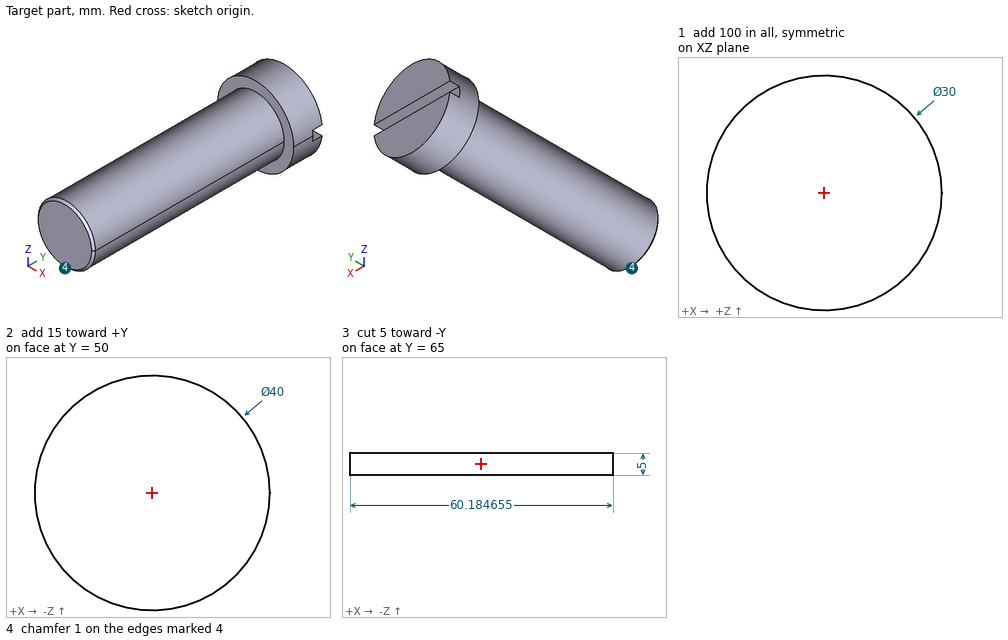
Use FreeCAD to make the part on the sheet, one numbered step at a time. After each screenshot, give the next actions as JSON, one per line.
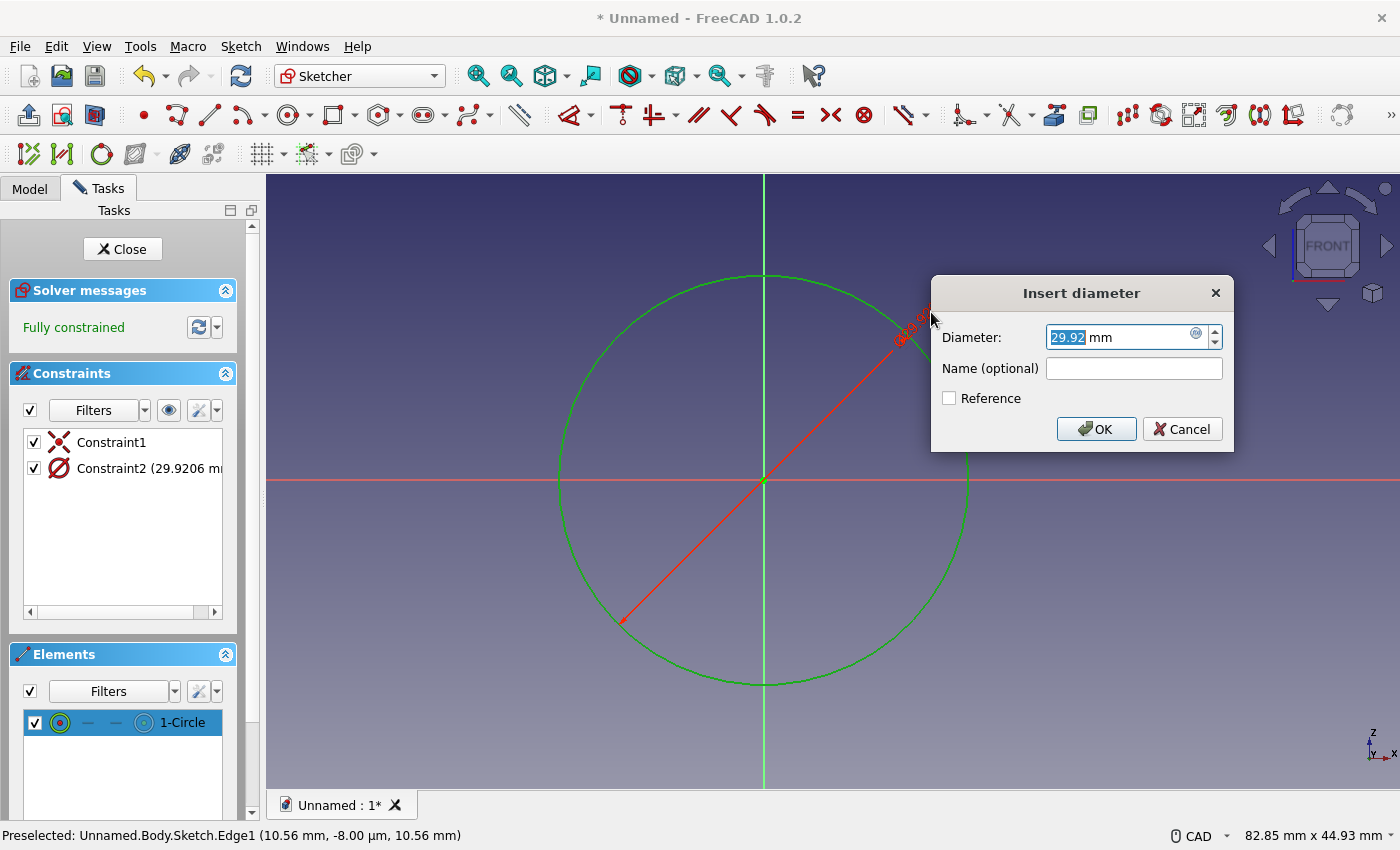
{"action": "type", "text": "30"}
{"action": "key", "text": "Return"}
{"action": "key", "text": "Escape"}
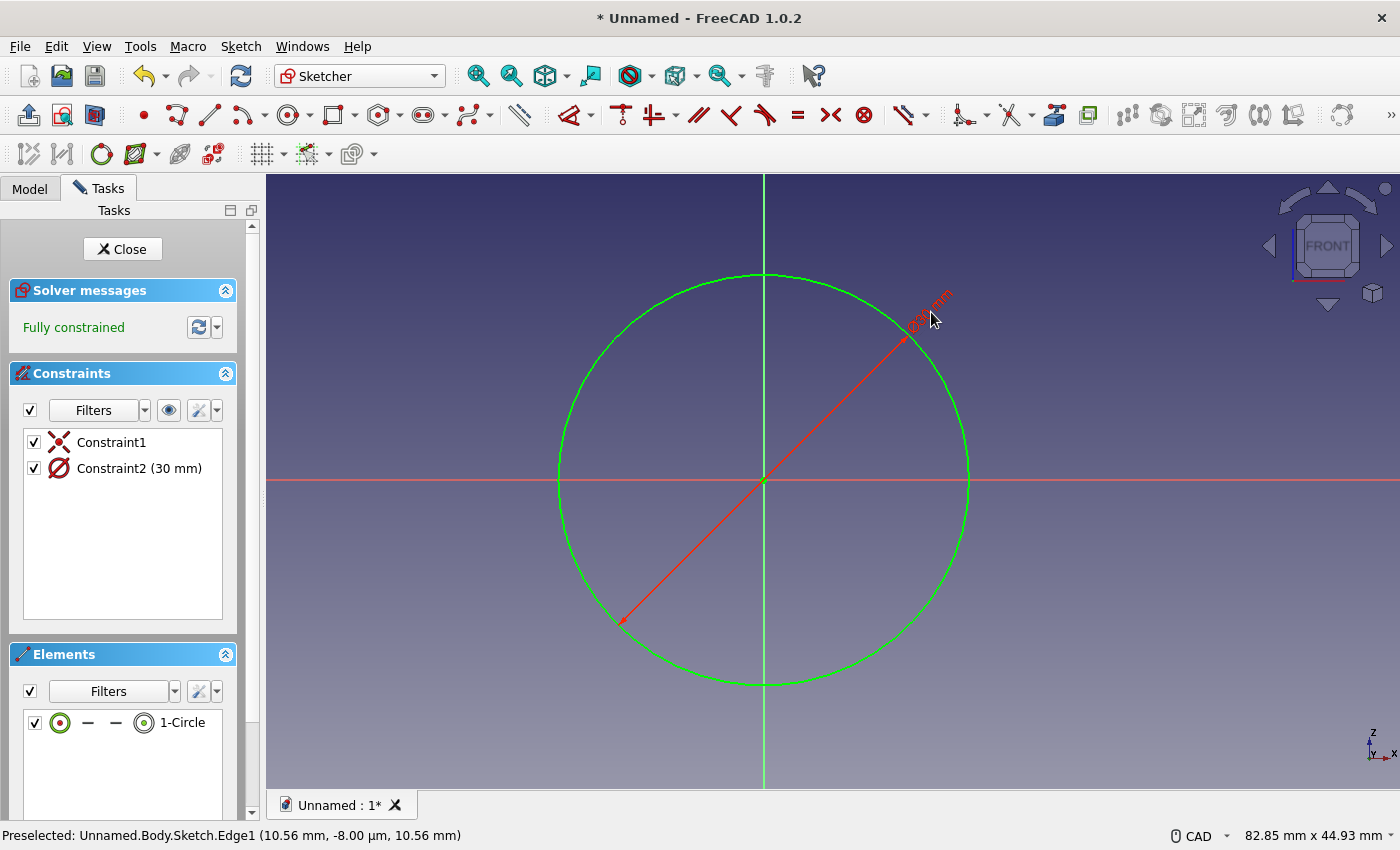
{"action": "left_click", "coordinate": [123, 249]}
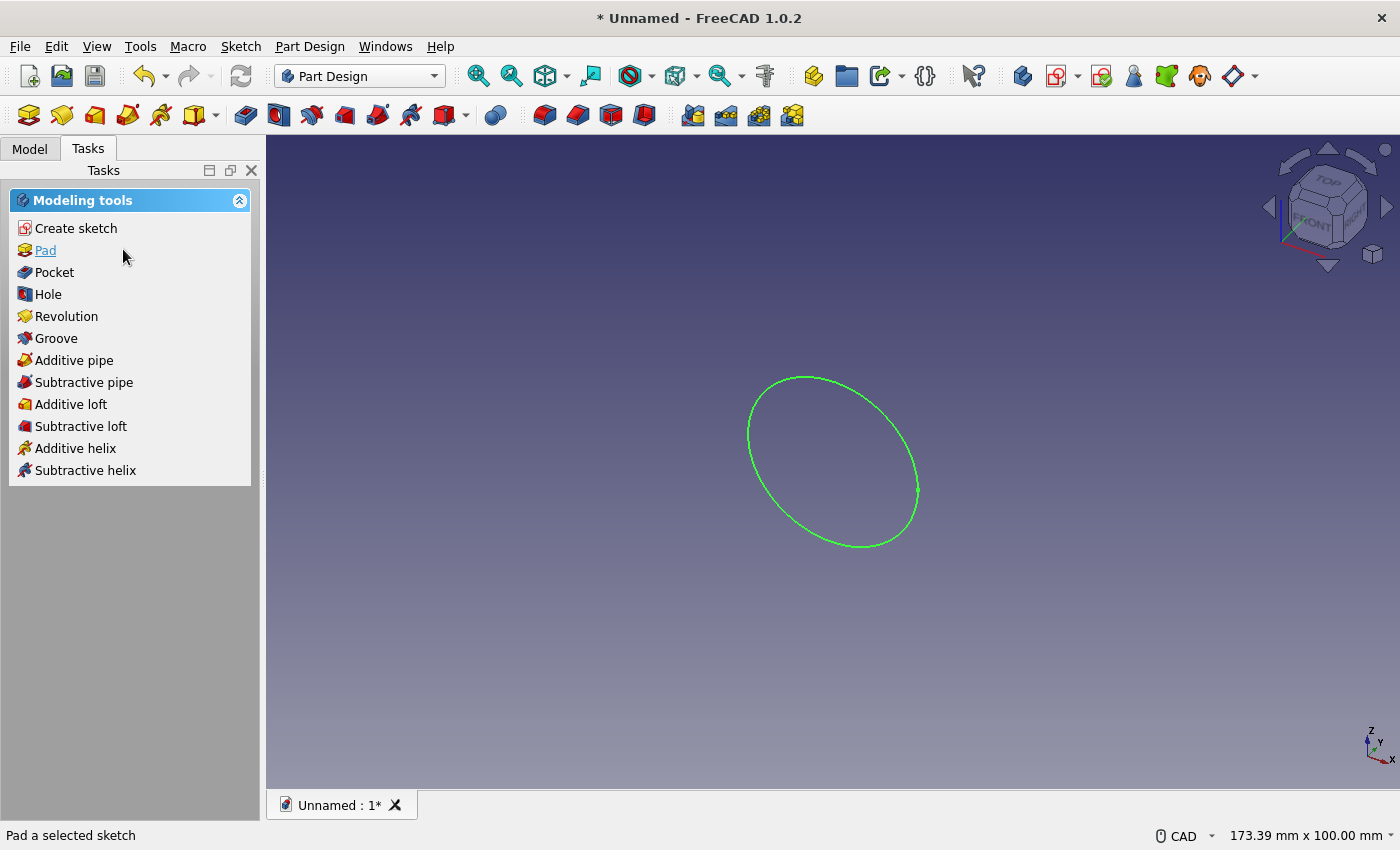
{"action": "left_click", "coordinate": [29, 116]}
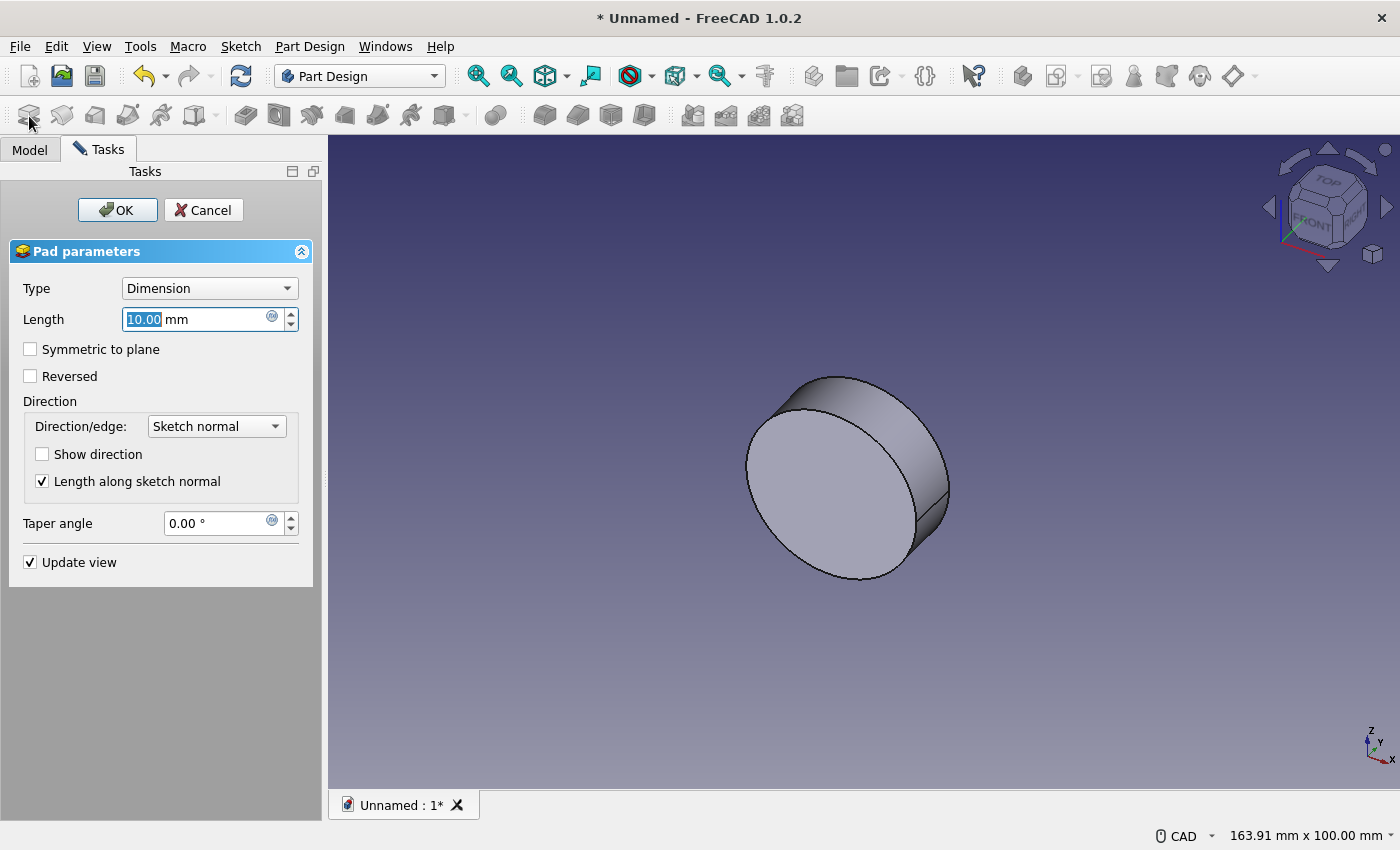
{"action": "type", "text": "100"}
{"action": "key", "text": "Tab"}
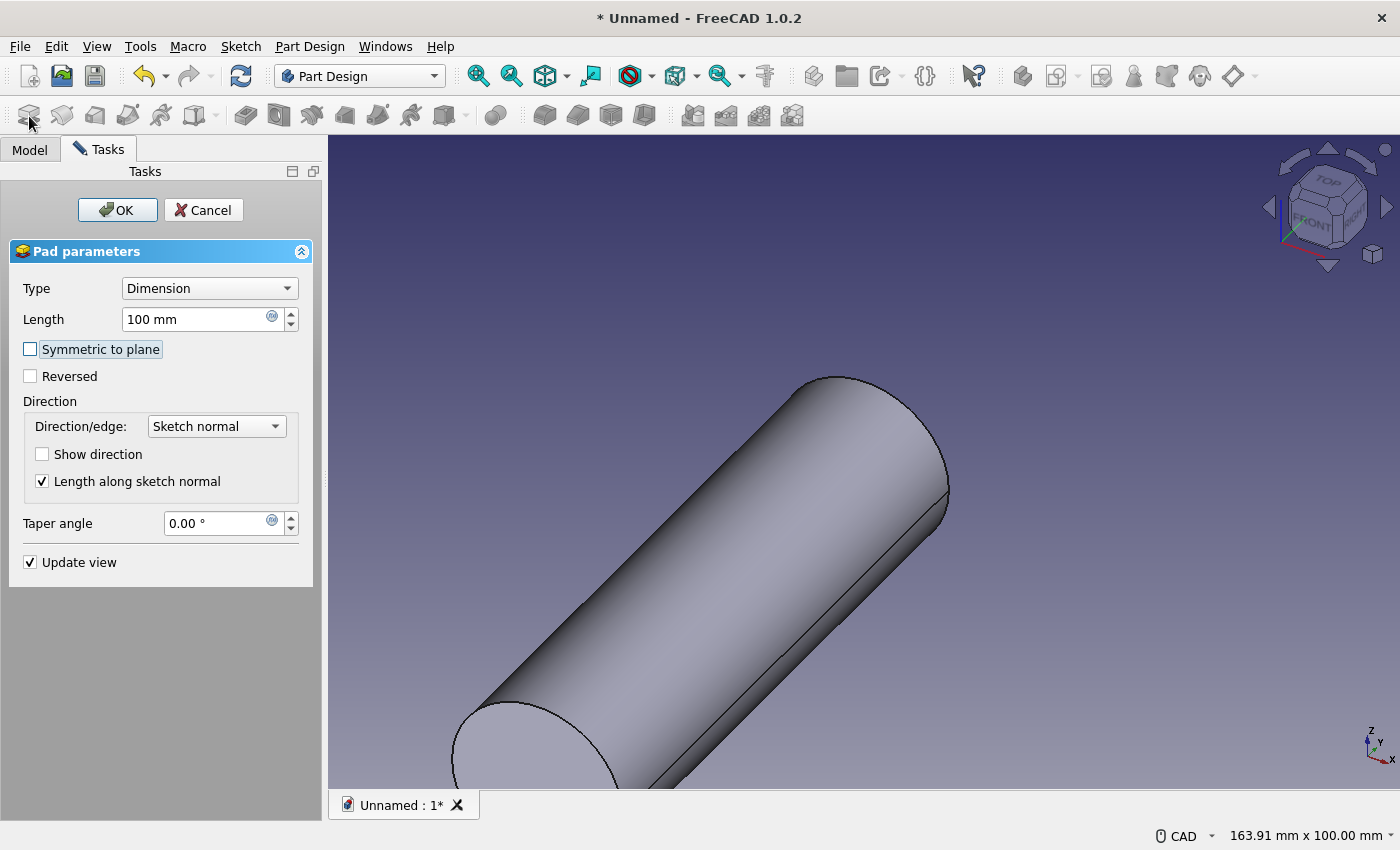
{"action": "left_click", "coordinate": [31, 349]}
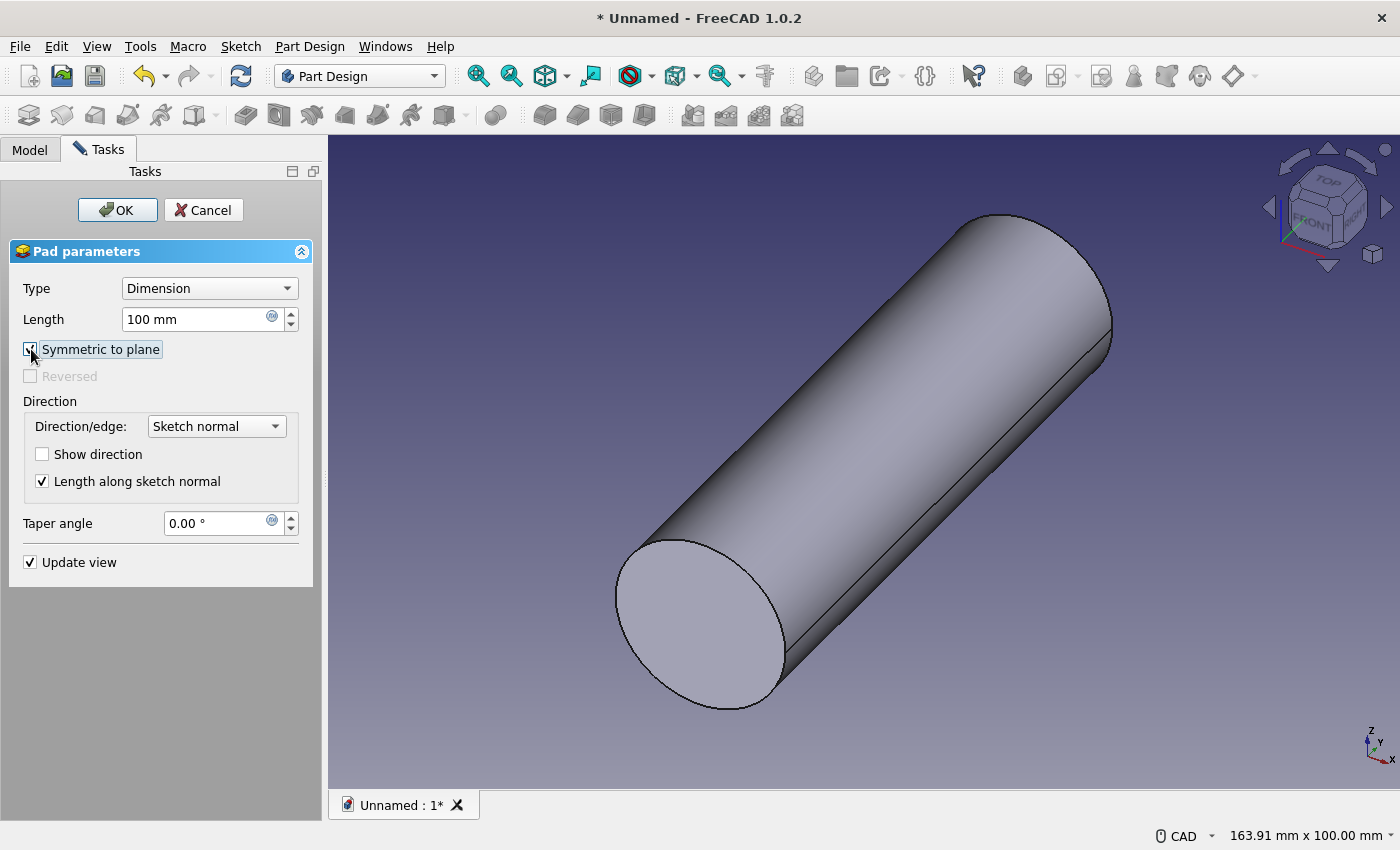
{"action": "left_click", "coordinate": [118, 210]}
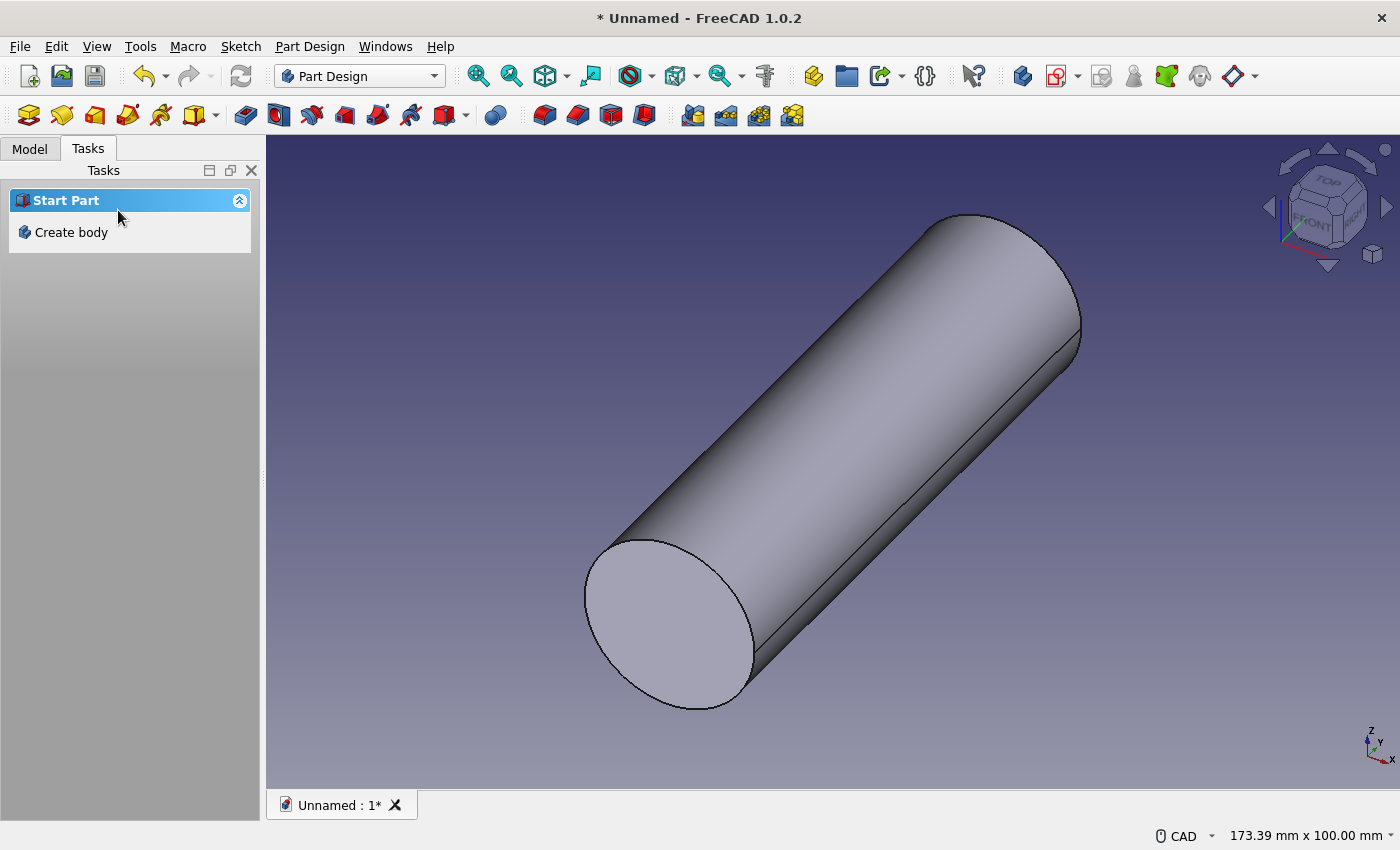
{"action": "key", "text": "4"}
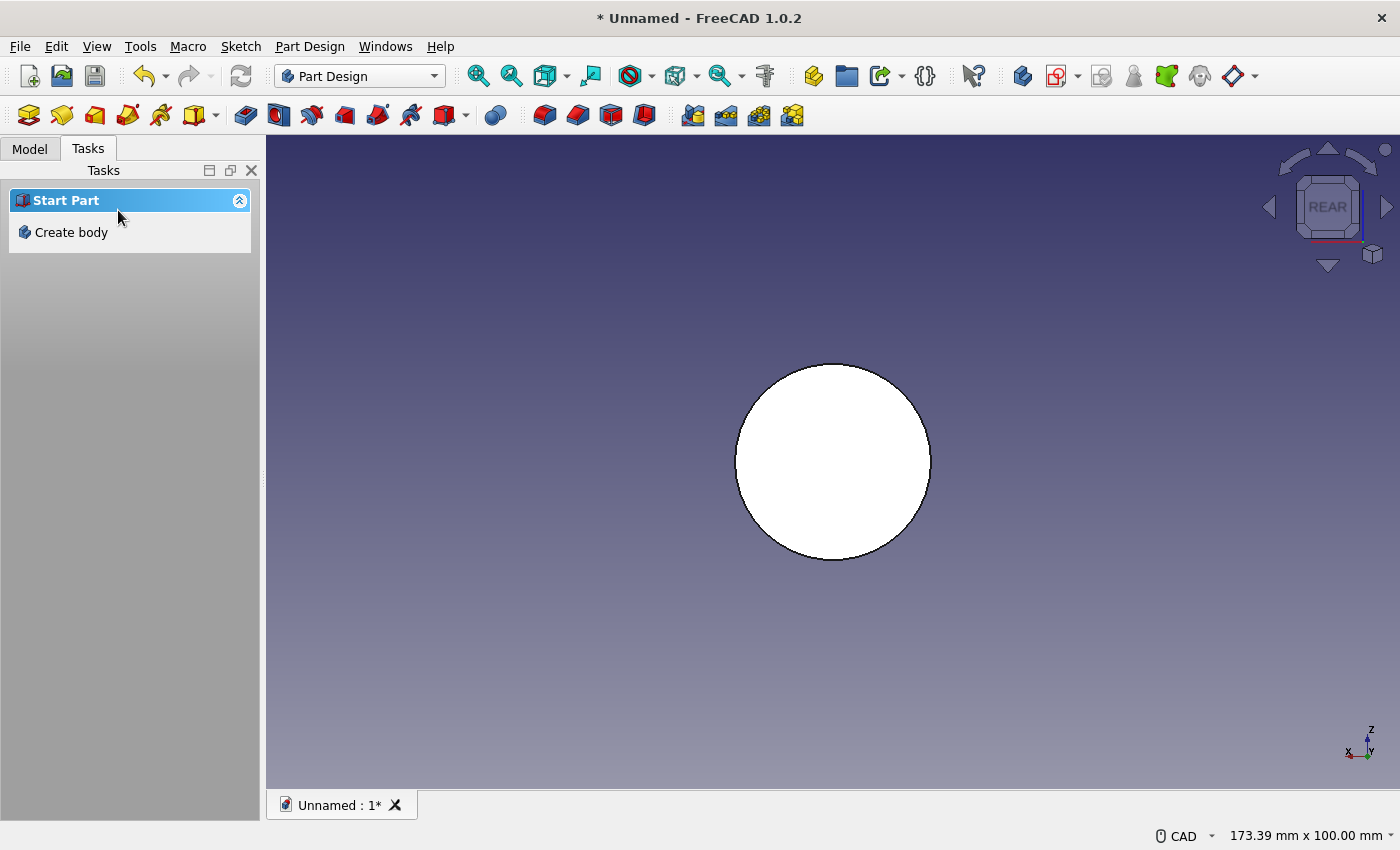
{"action": "left_click", "coordinate": [479, 76]}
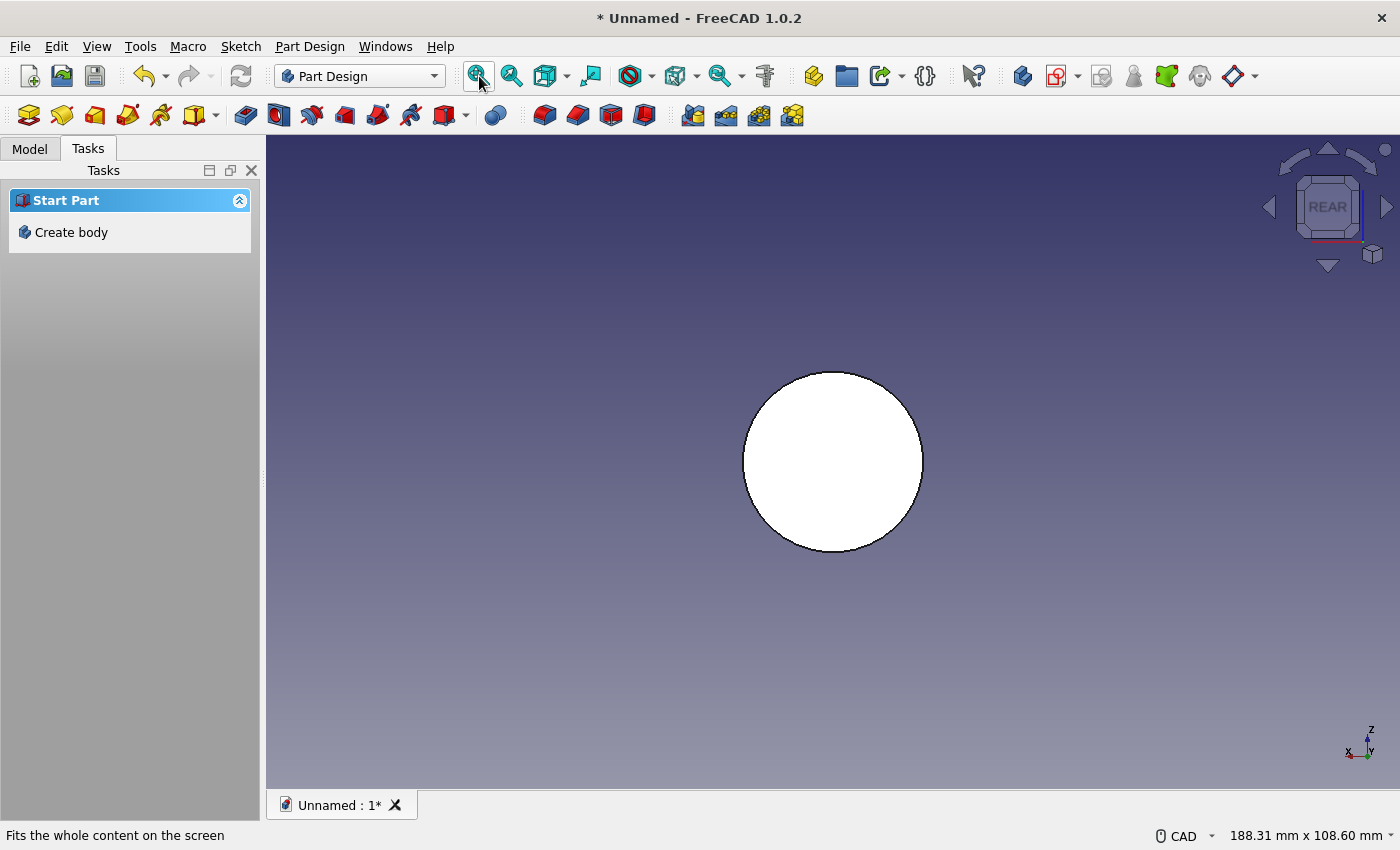
{"action": "left_click", "coordinate": [833, 461]}